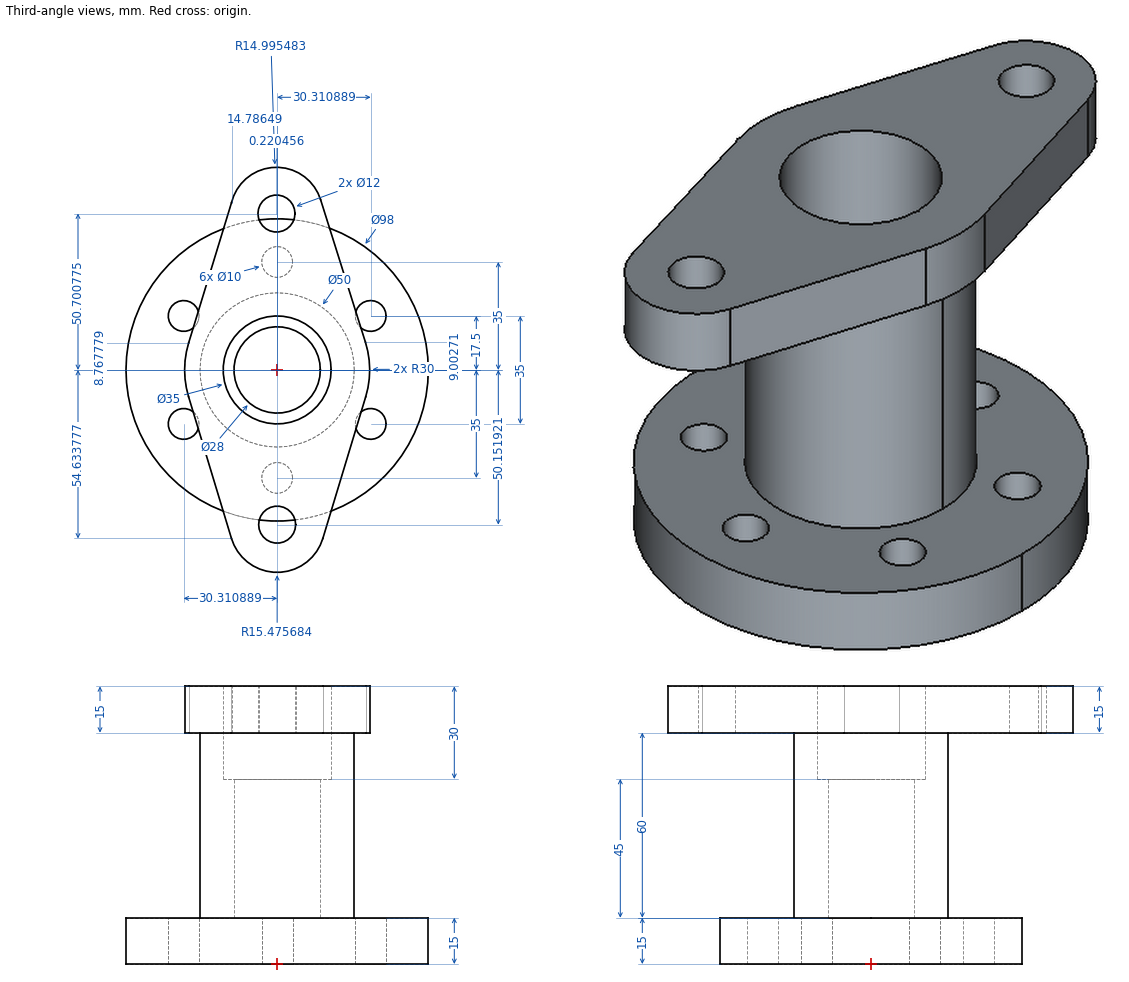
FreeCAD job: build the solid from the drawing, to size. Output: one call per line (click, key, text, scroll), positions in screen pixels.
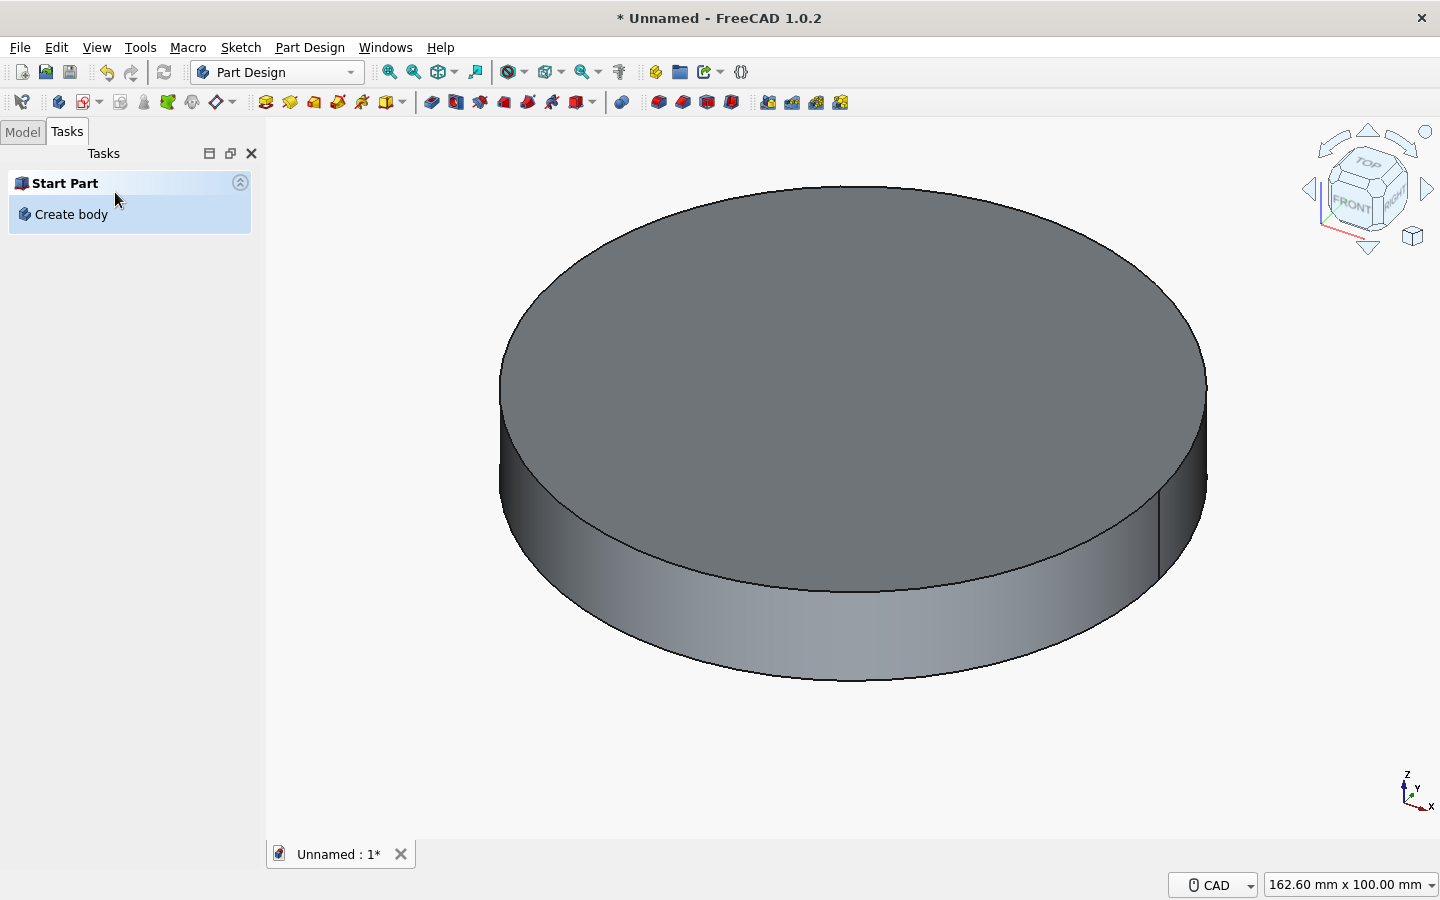
key(v)
key(f)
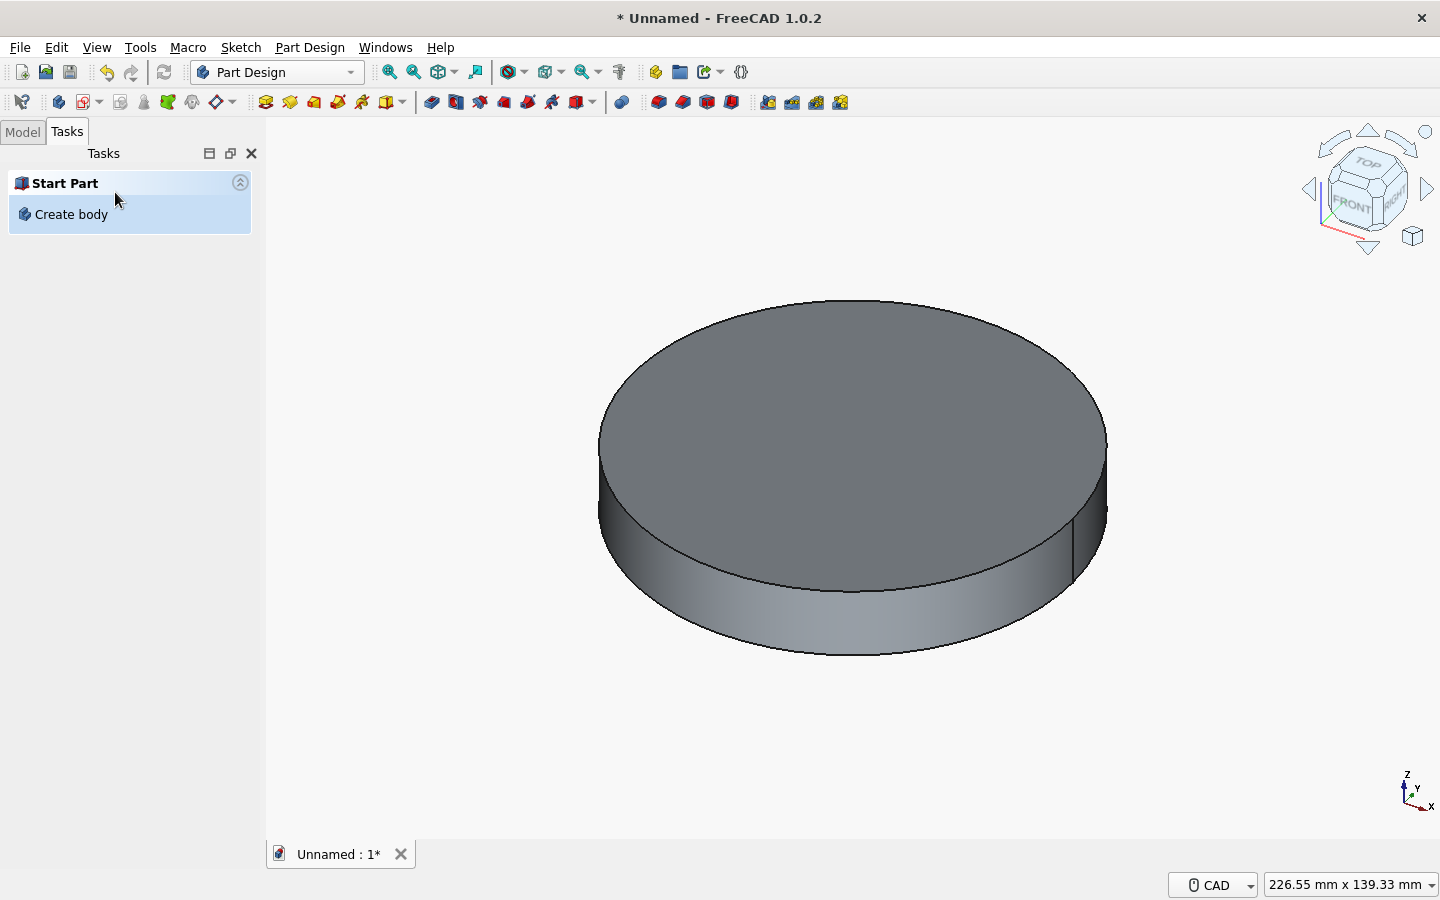
click(853, 445)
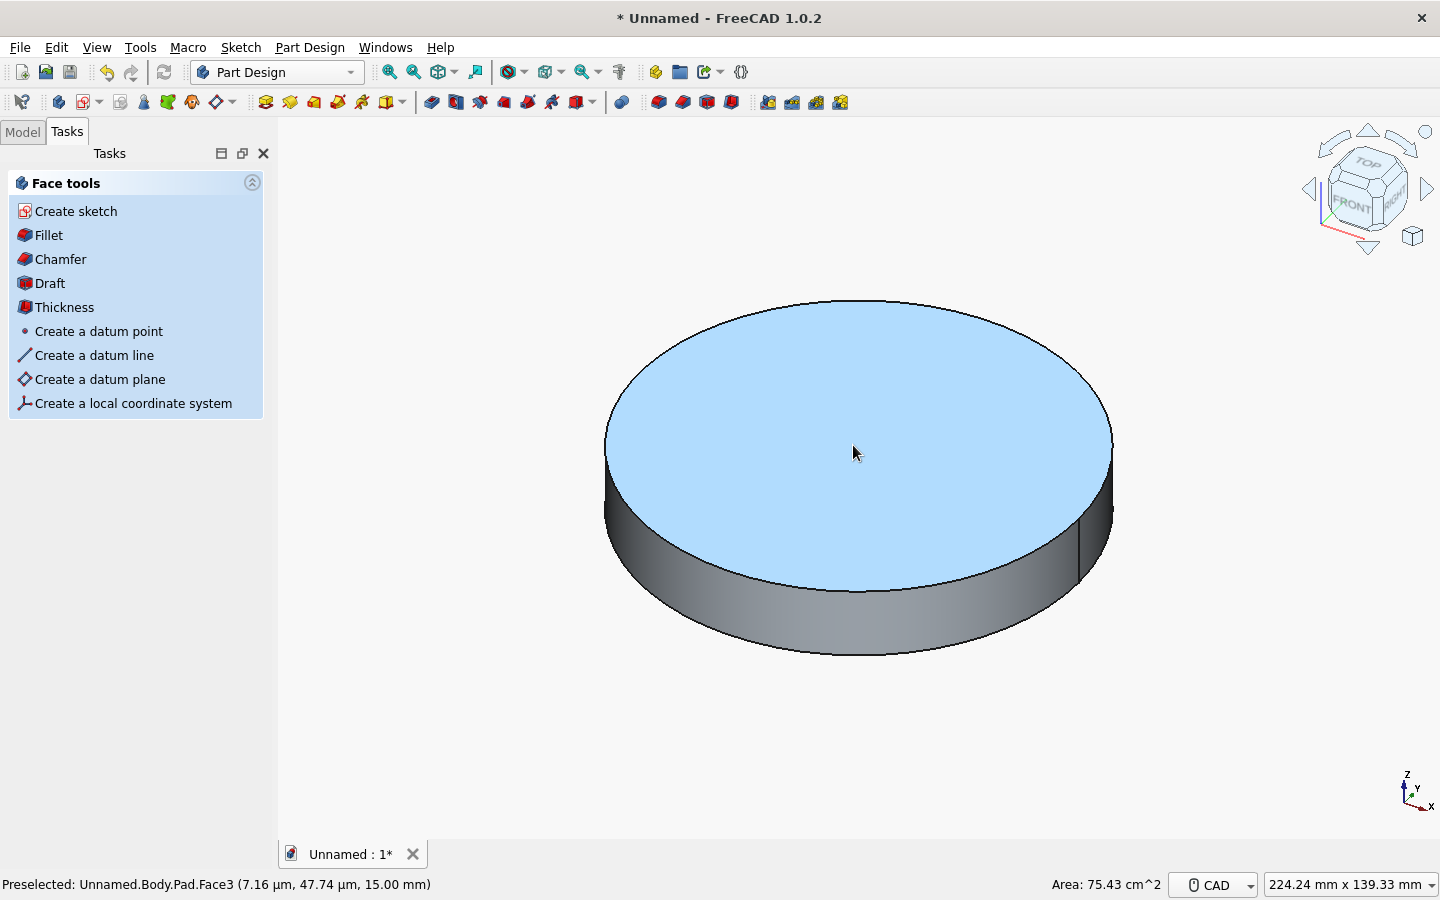
click(84, 102)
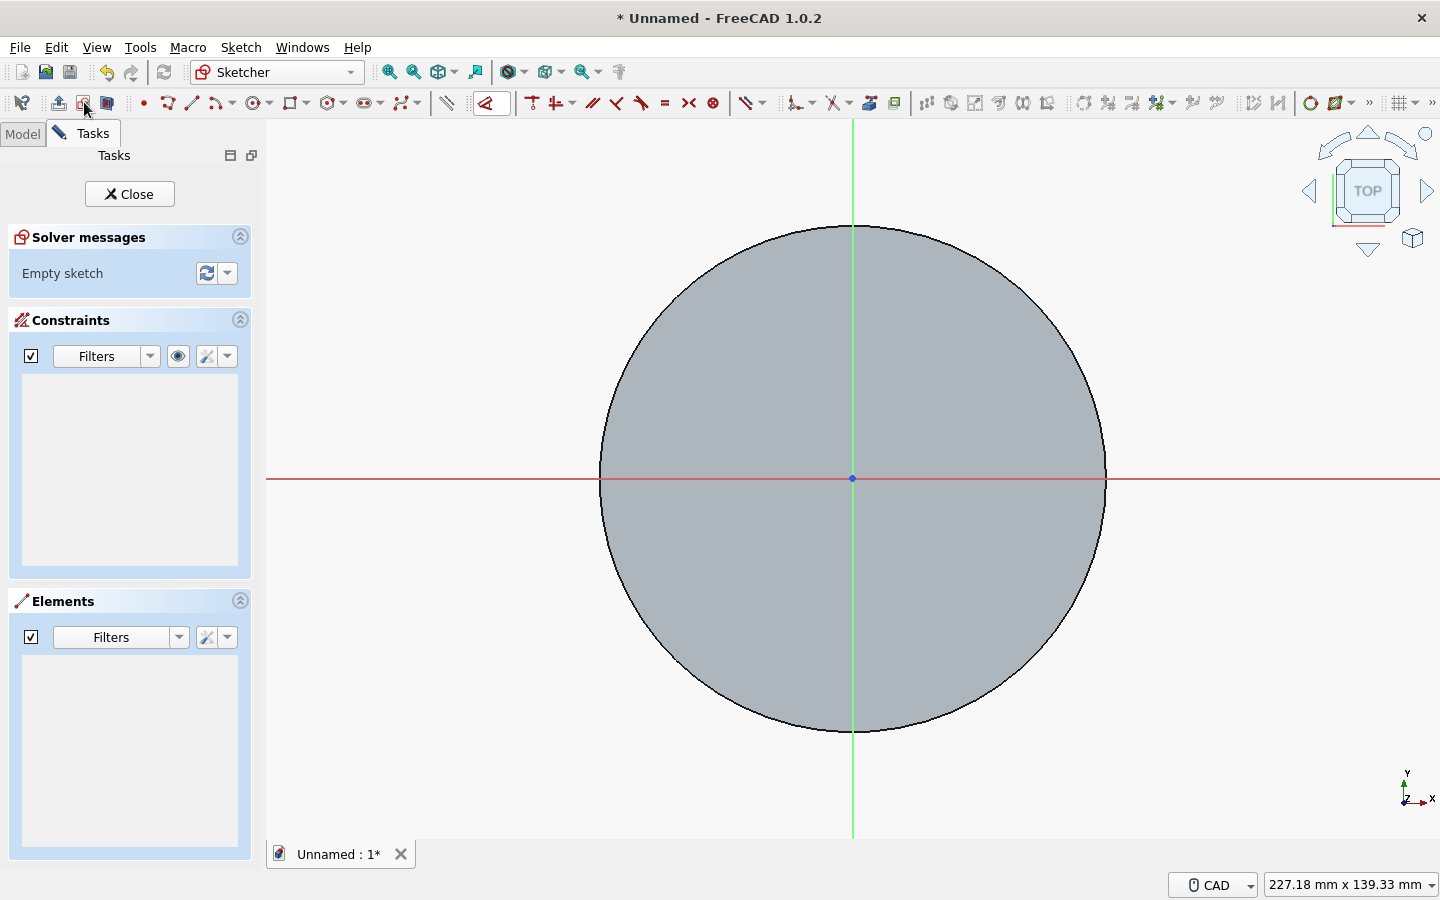
key(g)
key(c)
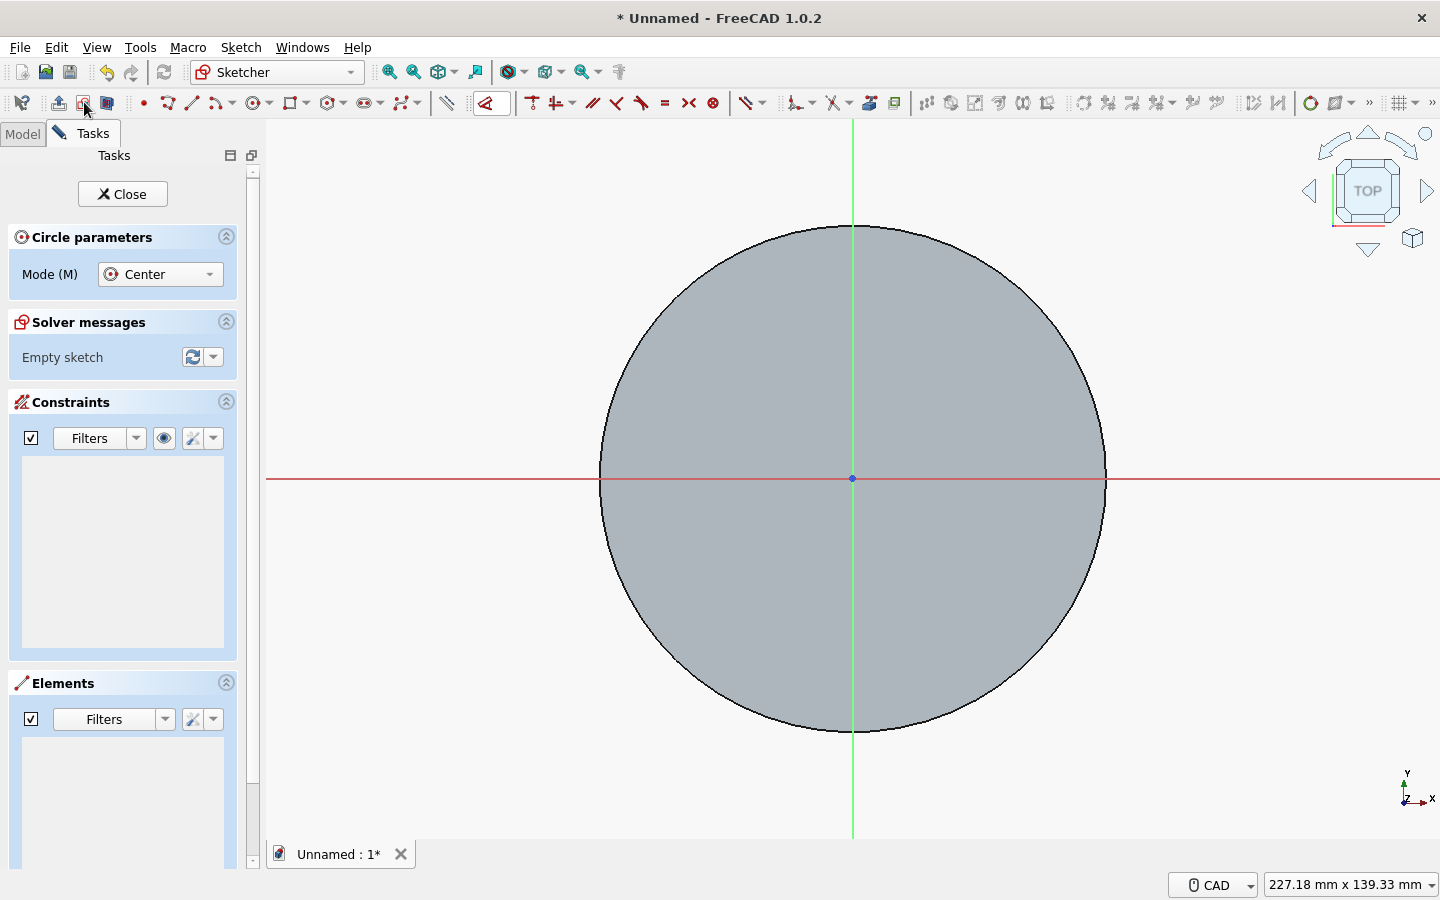
click(853, 298)
click(871, 280)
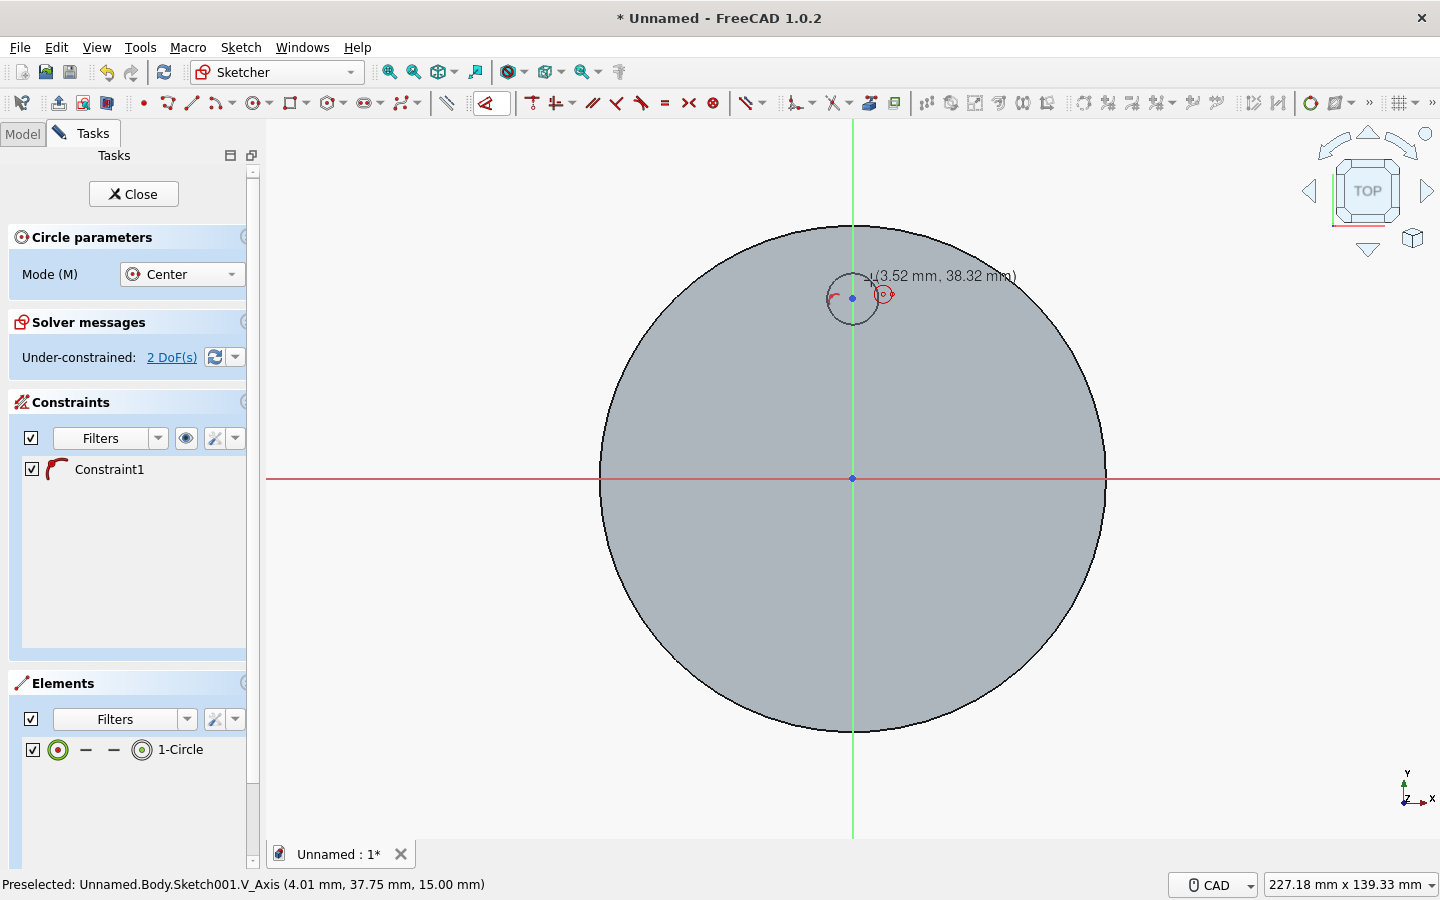
click(1009, 389)
click(1028, 370)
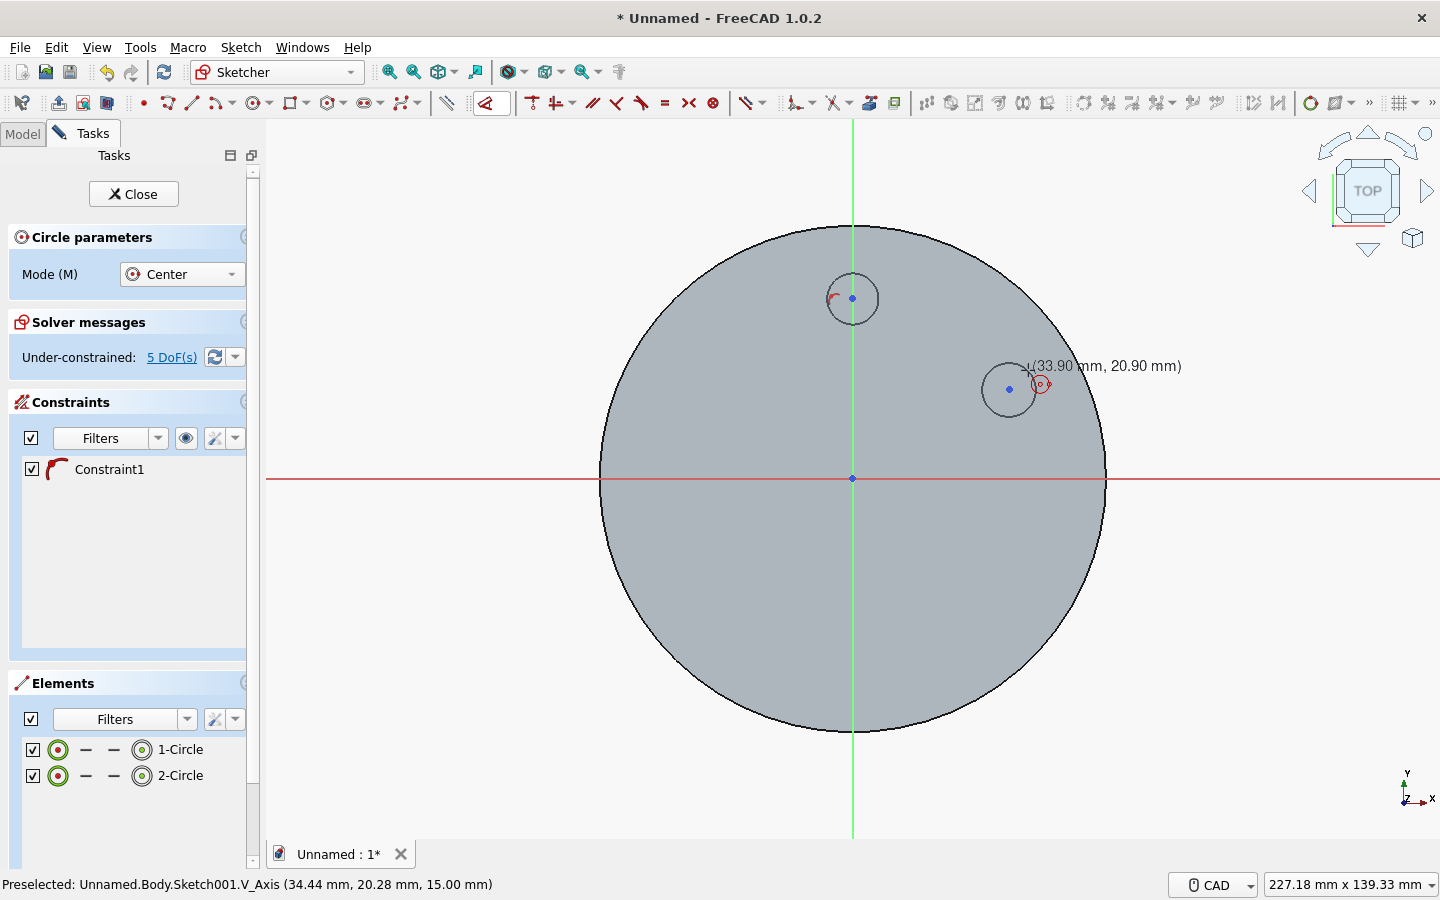
click(1009, 569)
click(1028, 551)